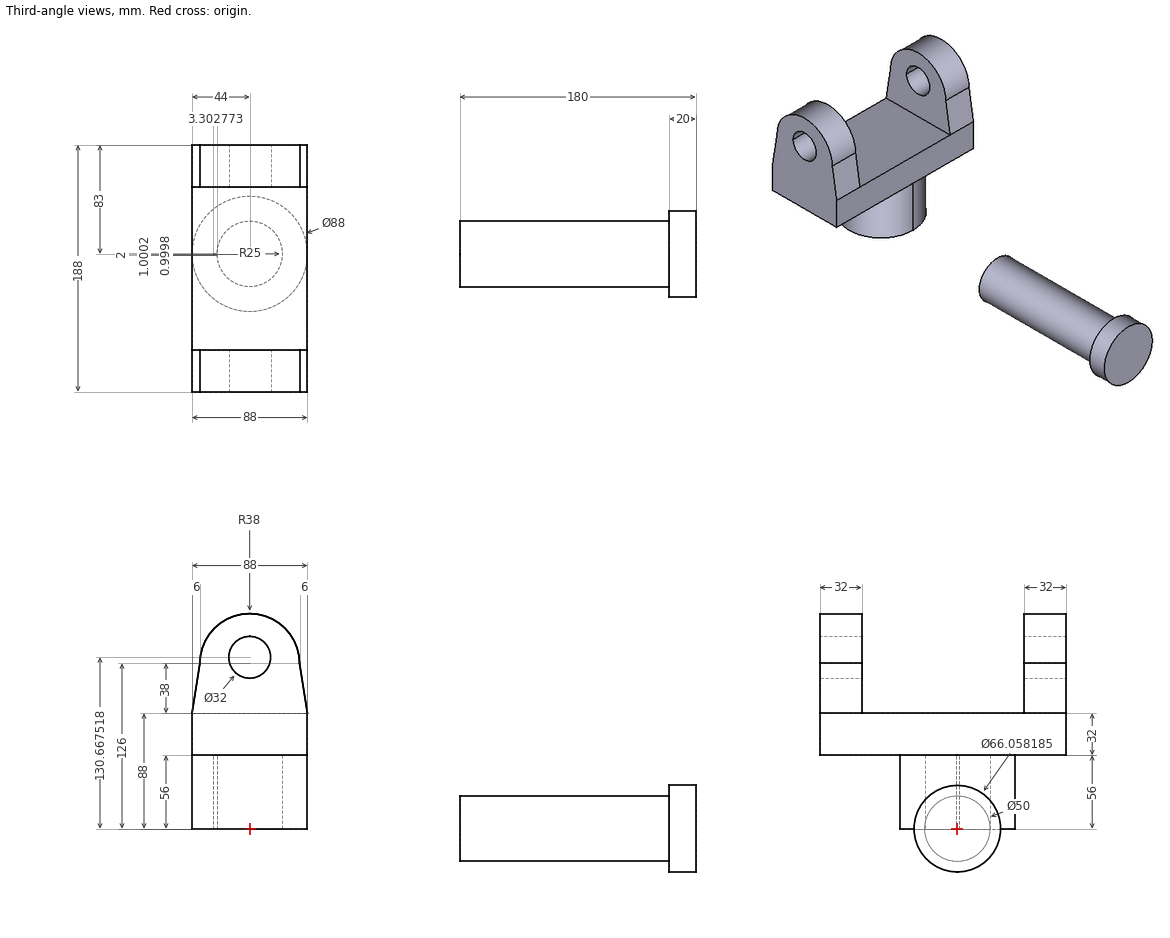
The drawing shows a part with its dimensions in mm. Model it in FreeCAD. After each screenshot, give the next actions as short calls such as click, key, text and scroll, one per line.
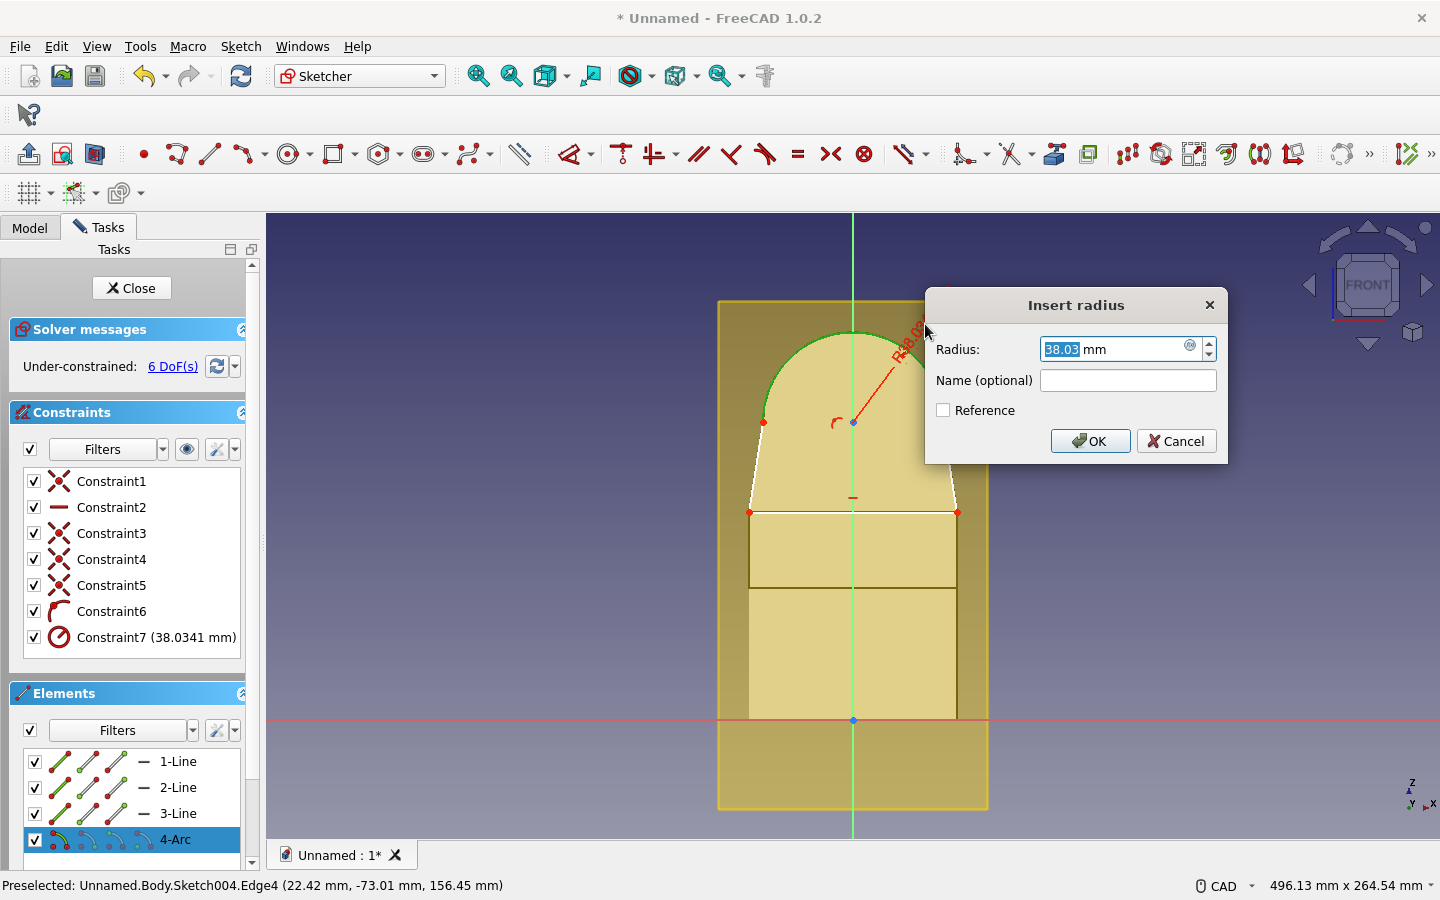
text(38)
key(Return)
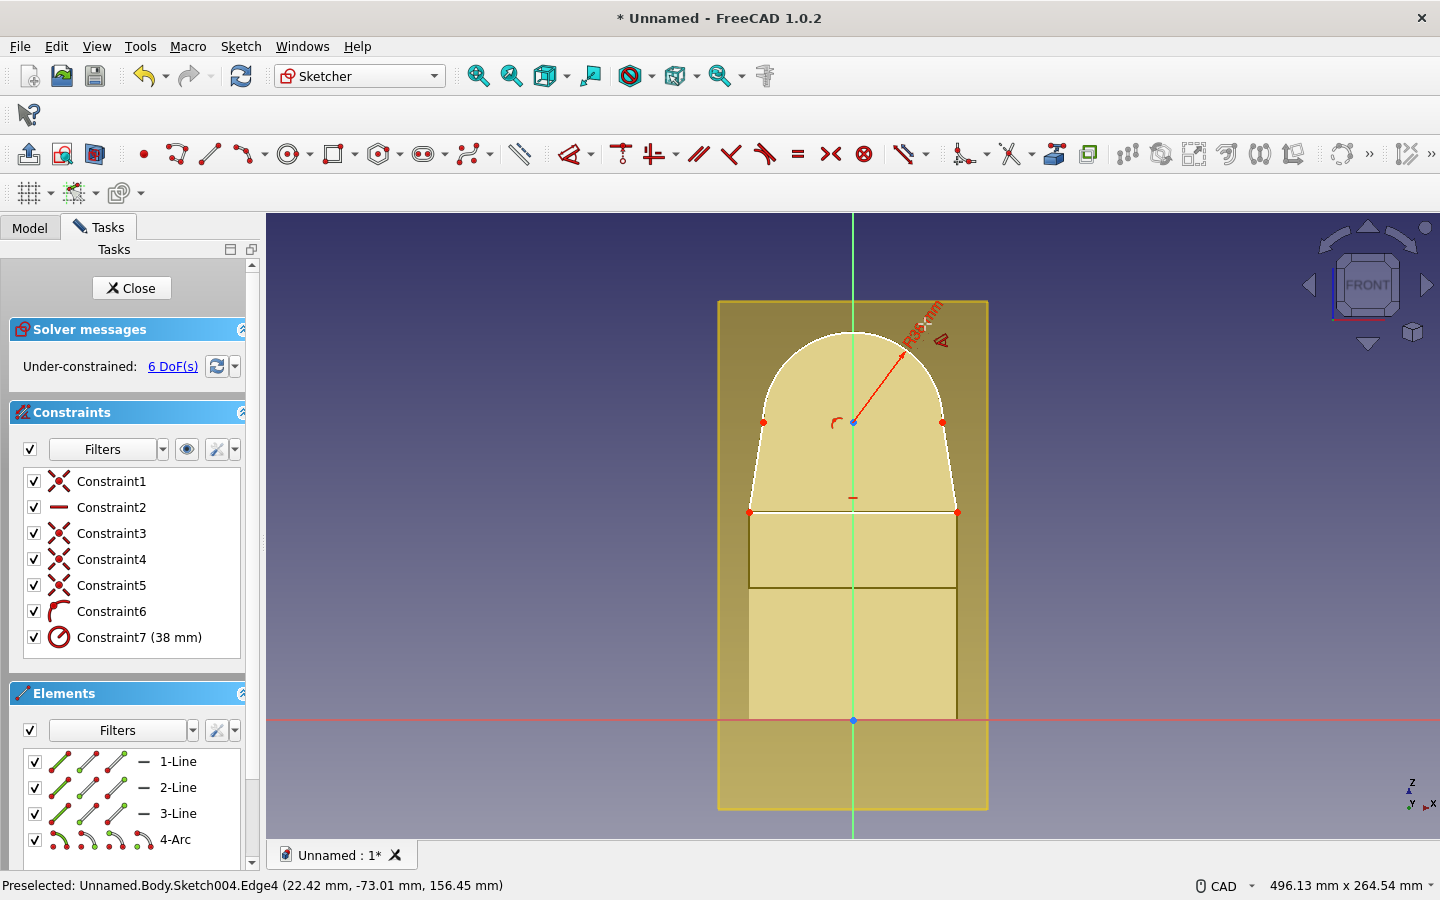
click(811, 513)
click(805, 479)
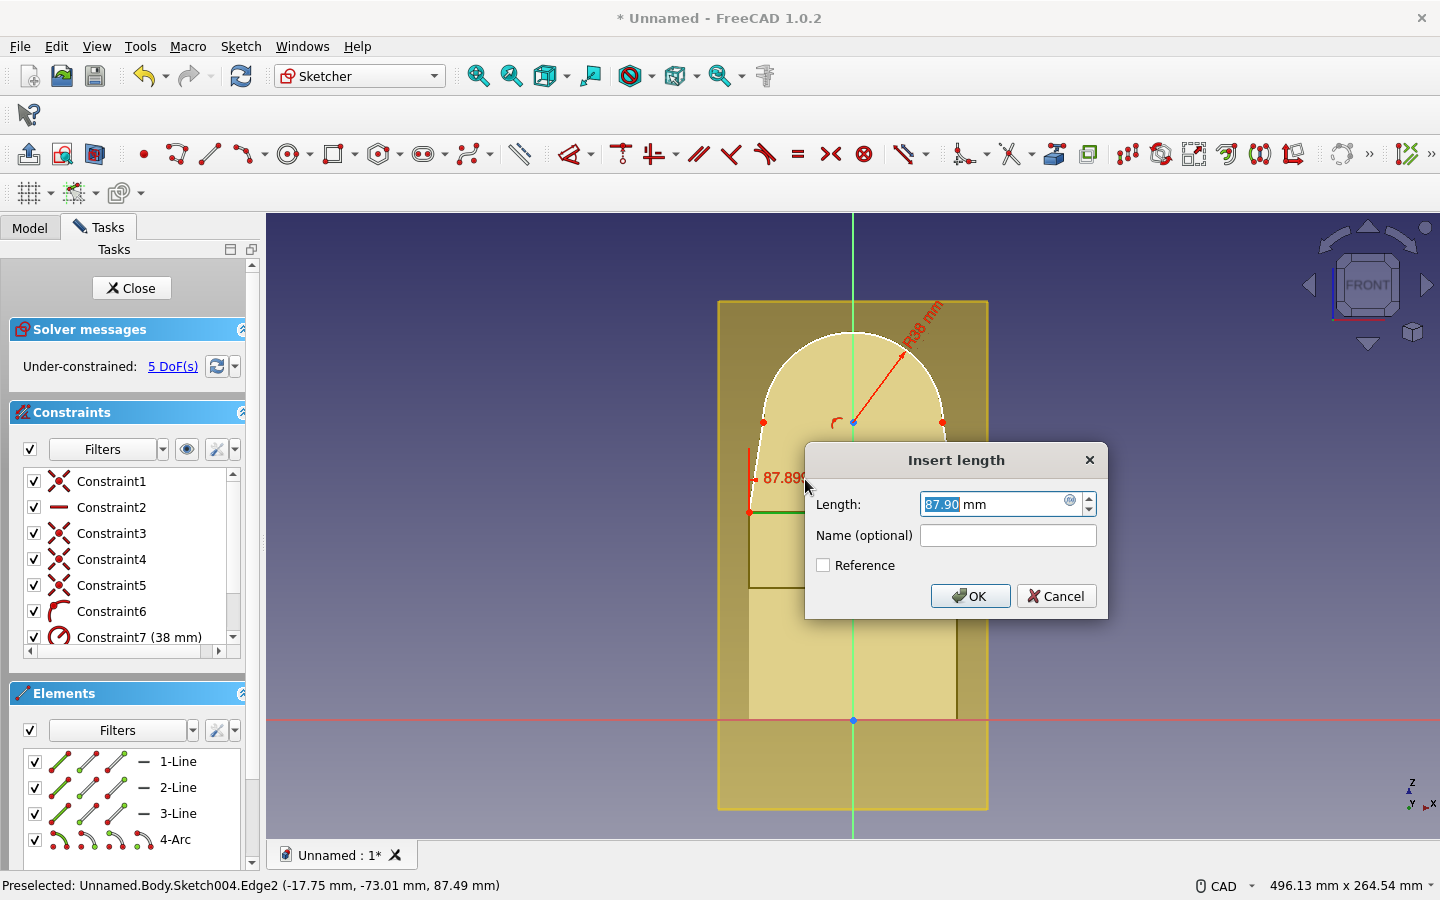
text(88)
key(Return)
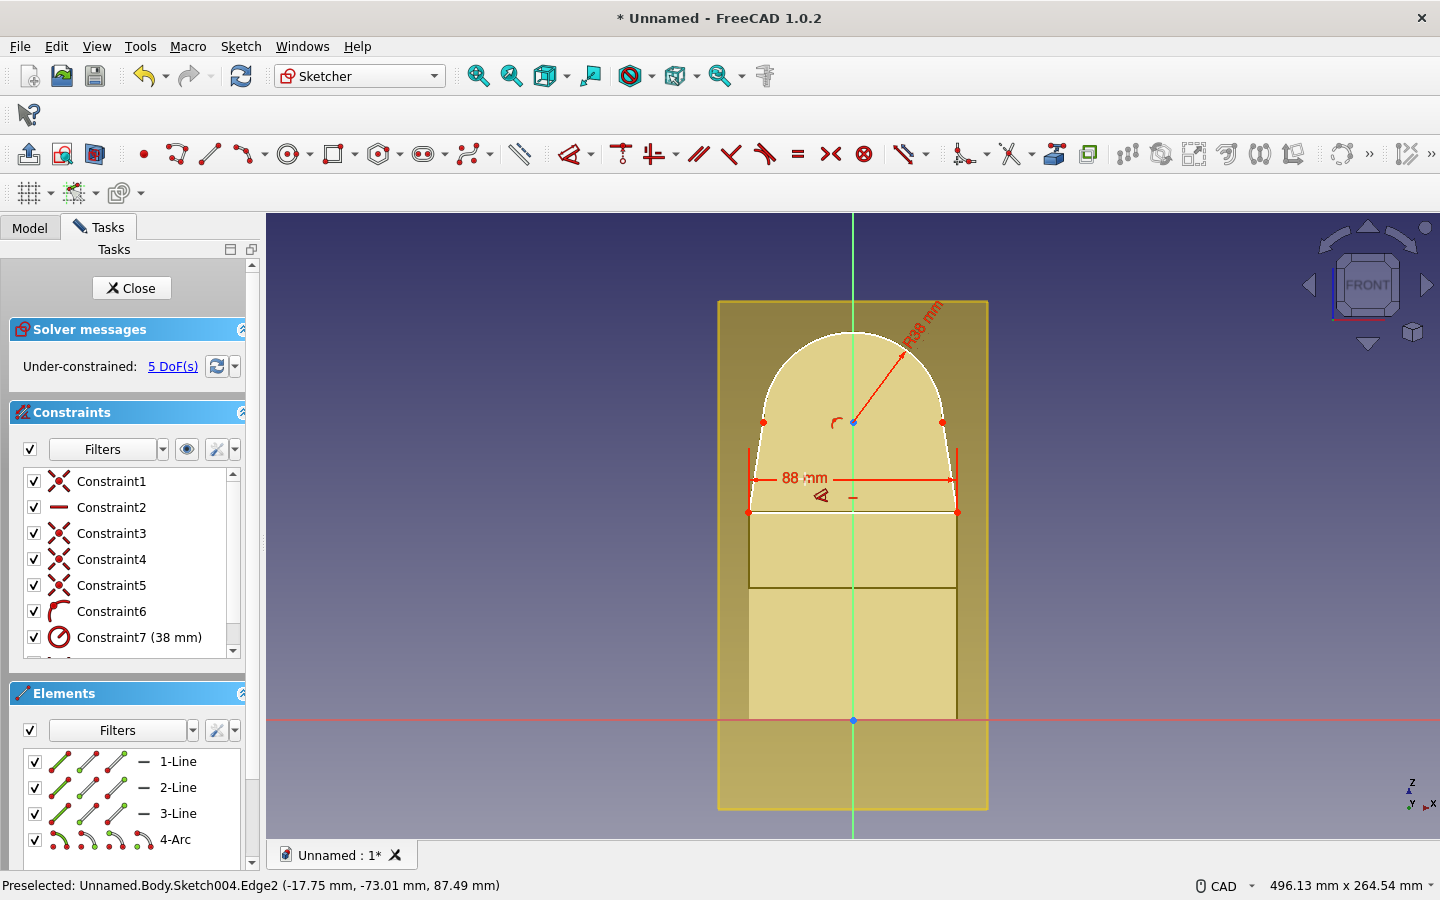
scroll(759, 450, up, 6)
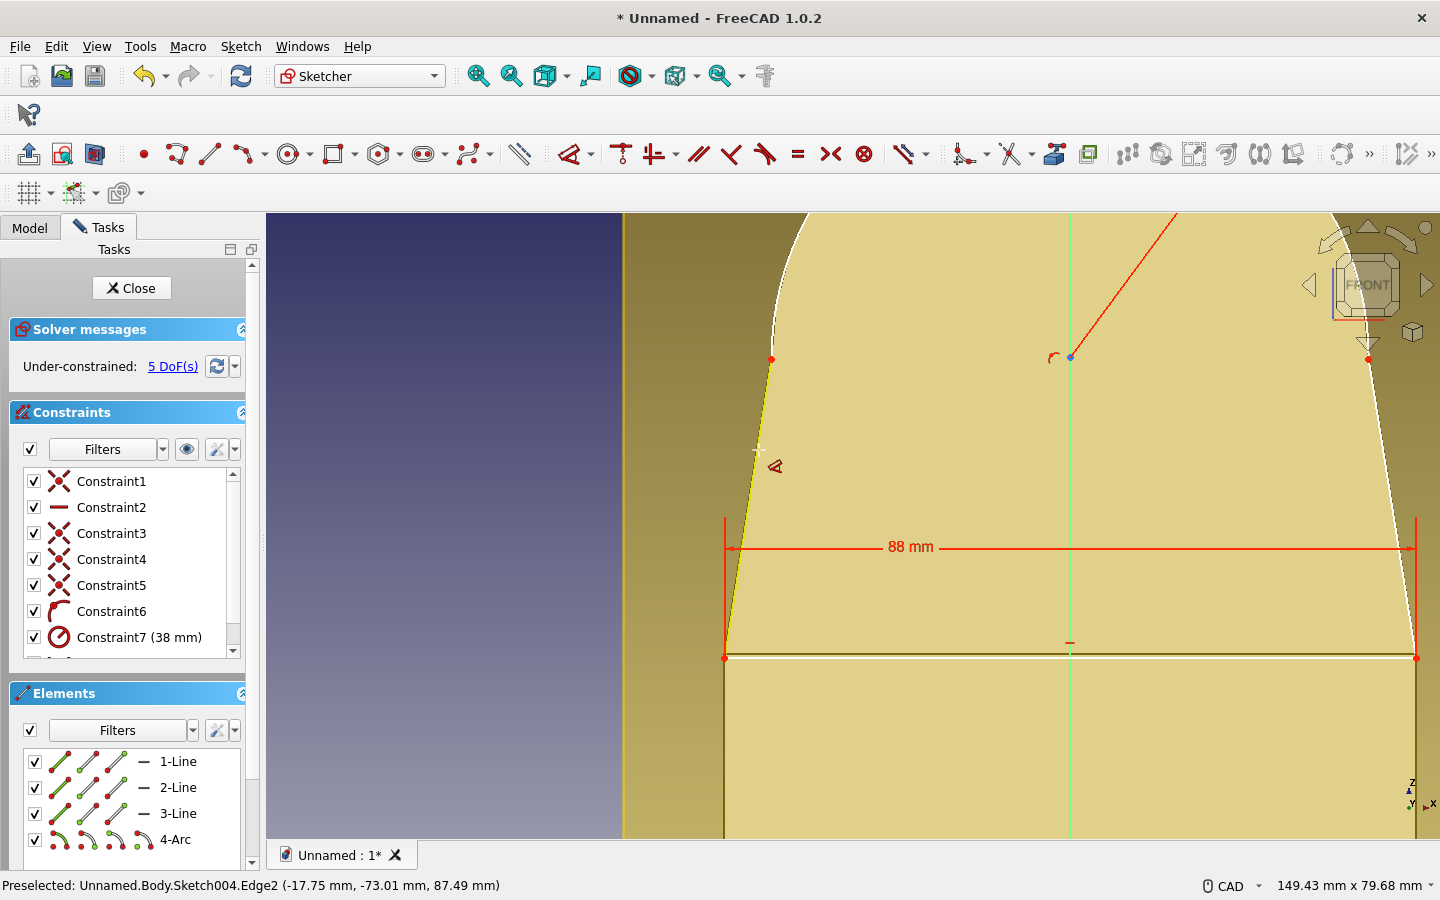
click(758, 449)
click(748, 325)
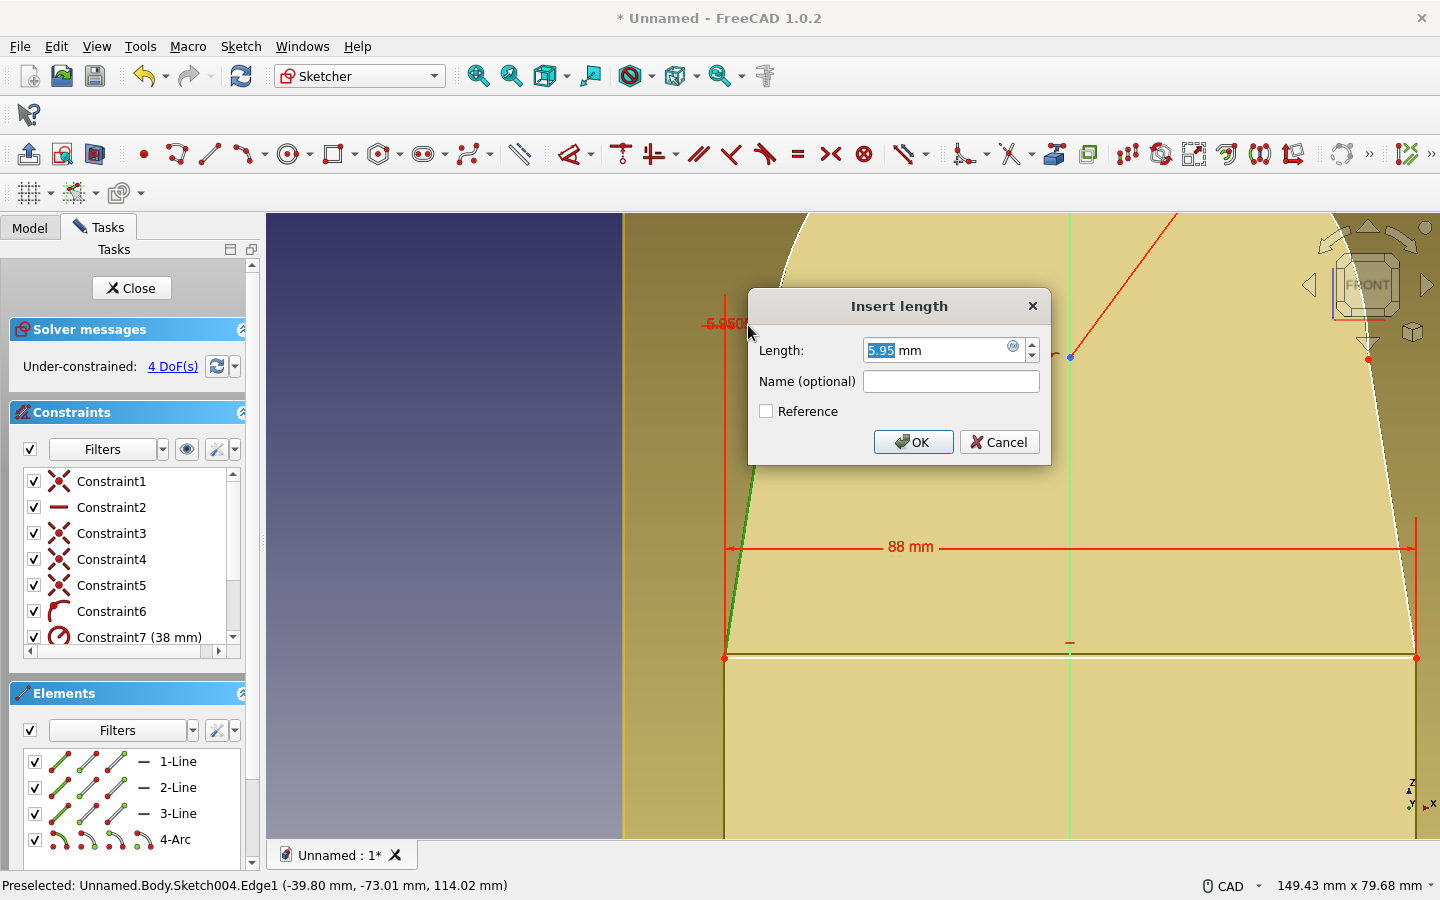
text(6)
key(Return)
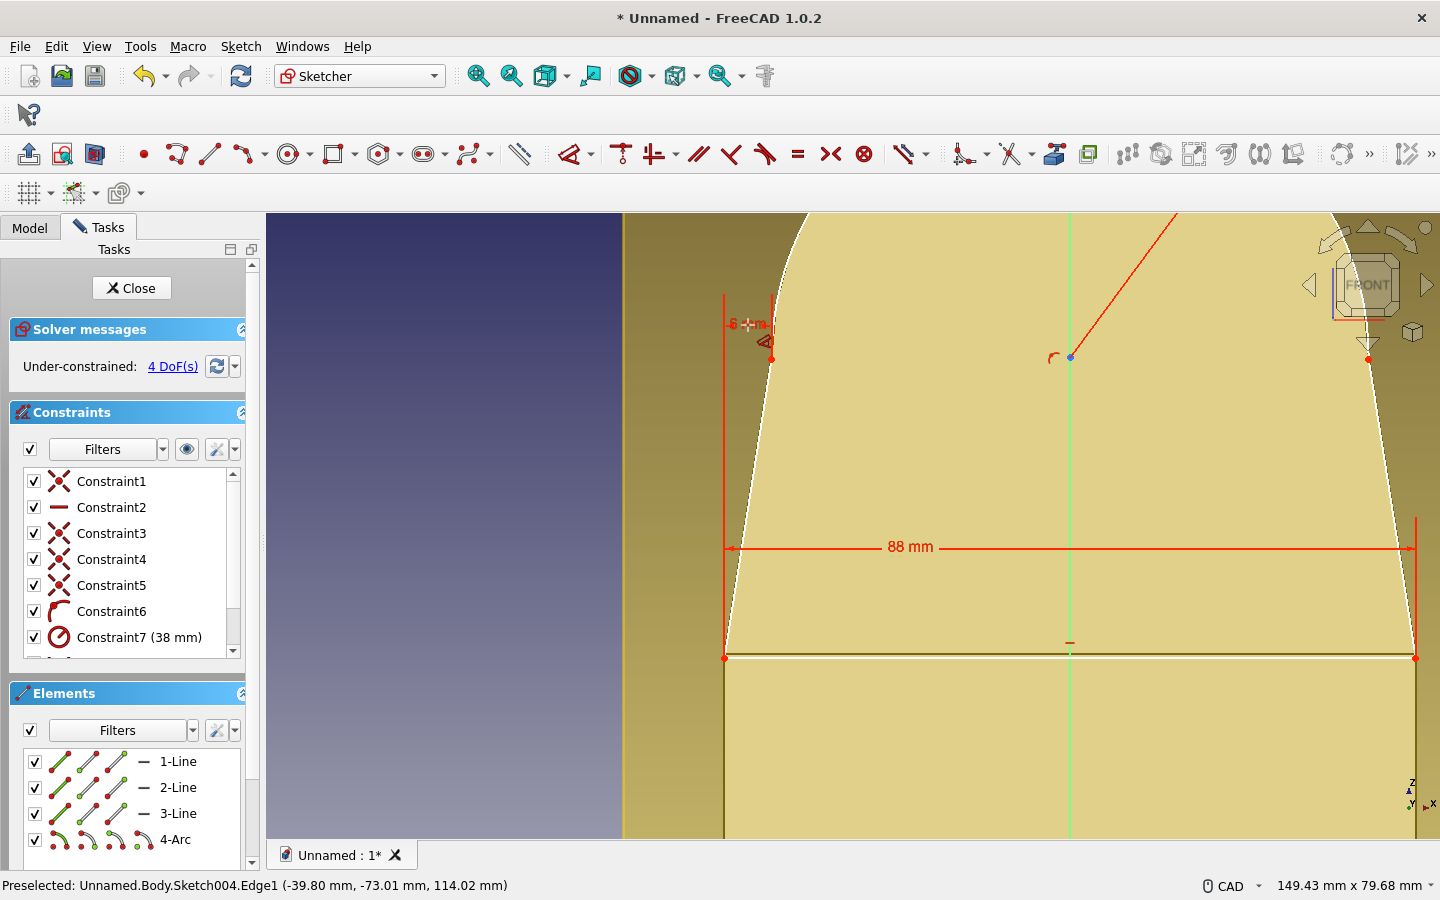
click(724, 658)
click(690, 735)